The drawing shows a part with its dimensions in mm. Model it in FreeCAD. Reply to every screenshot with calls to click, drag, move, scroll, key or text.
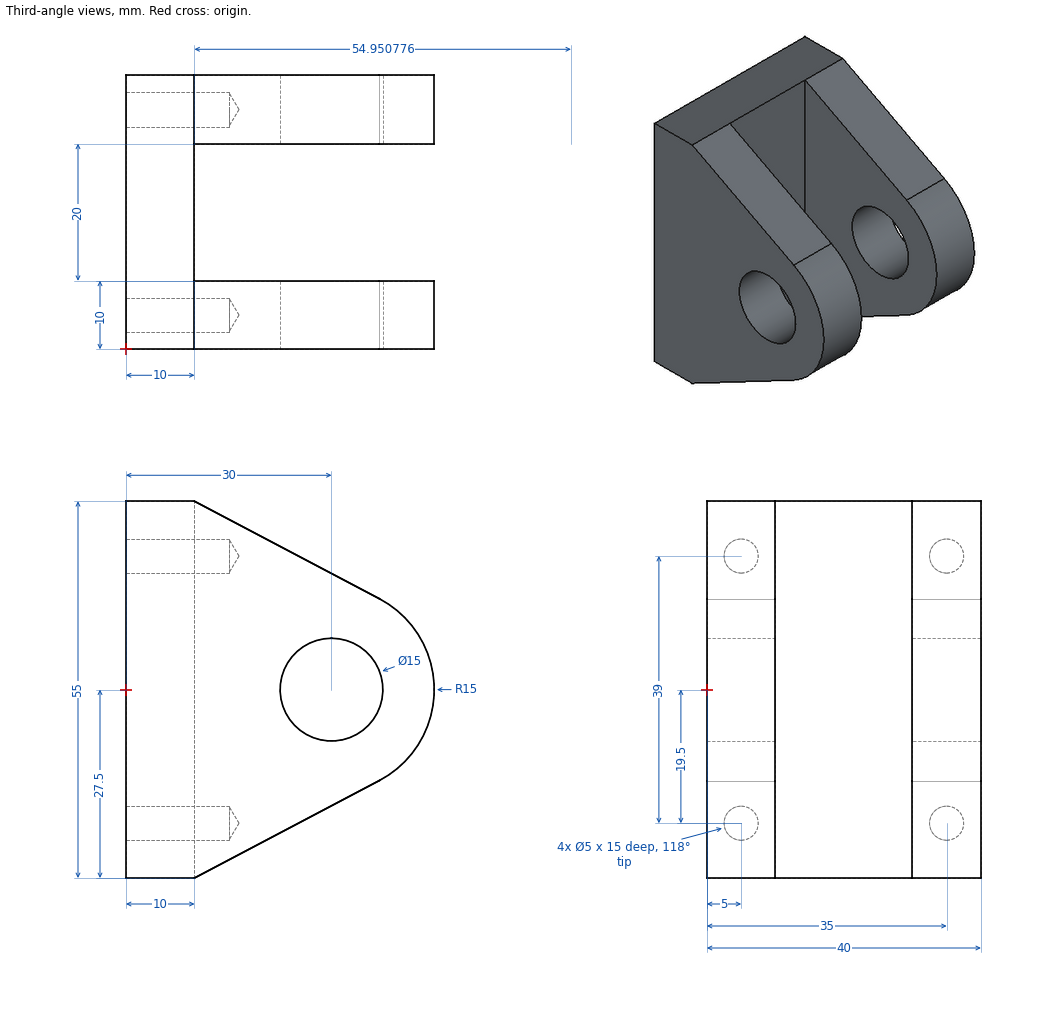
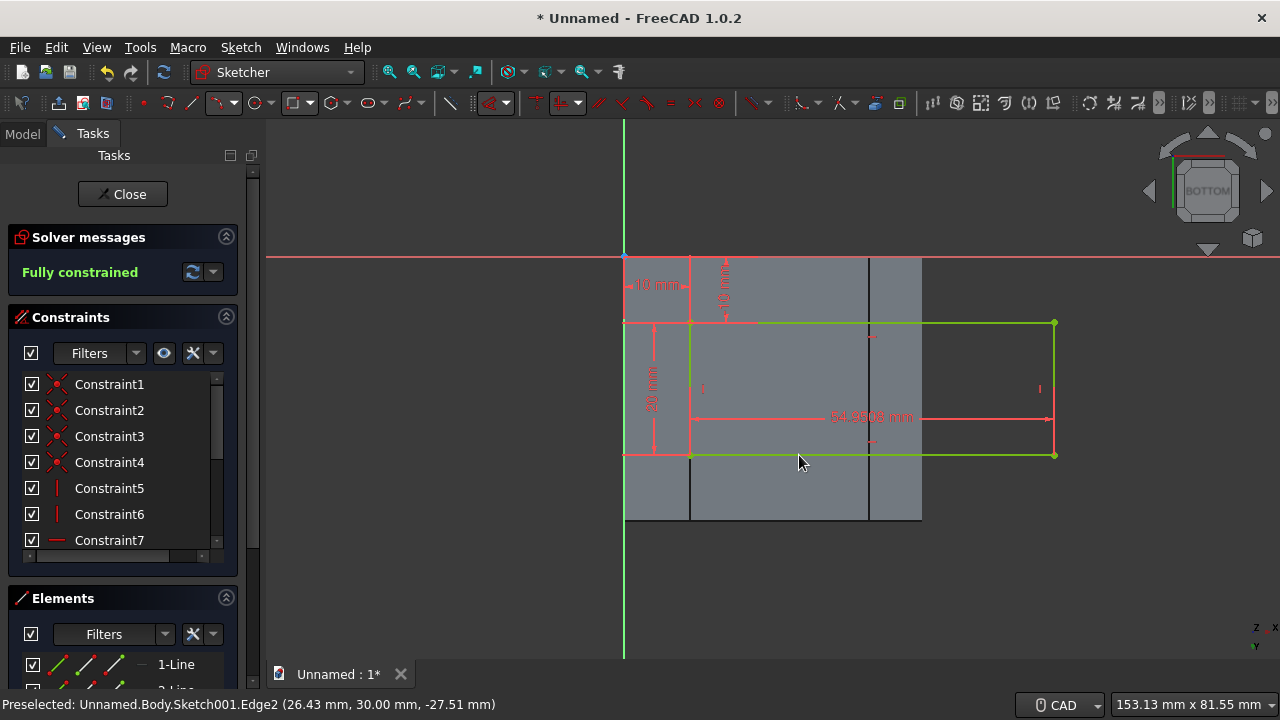
click(123, 194)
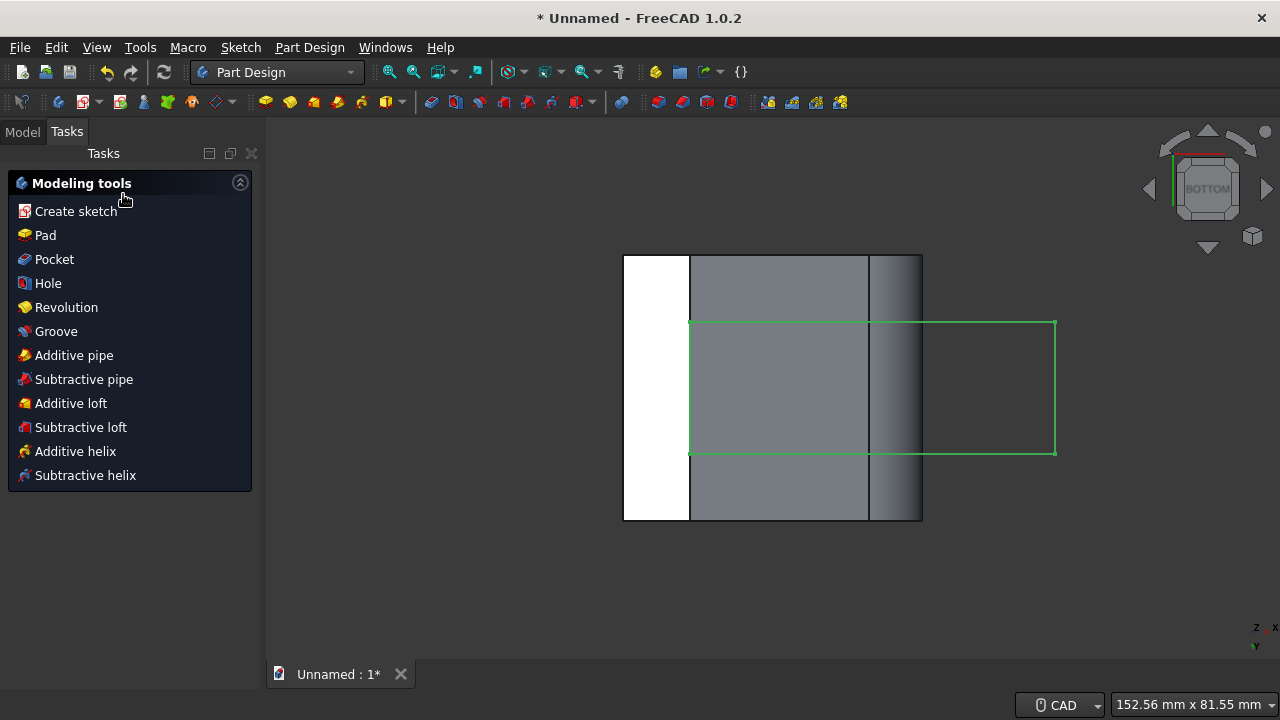
click(432, 102)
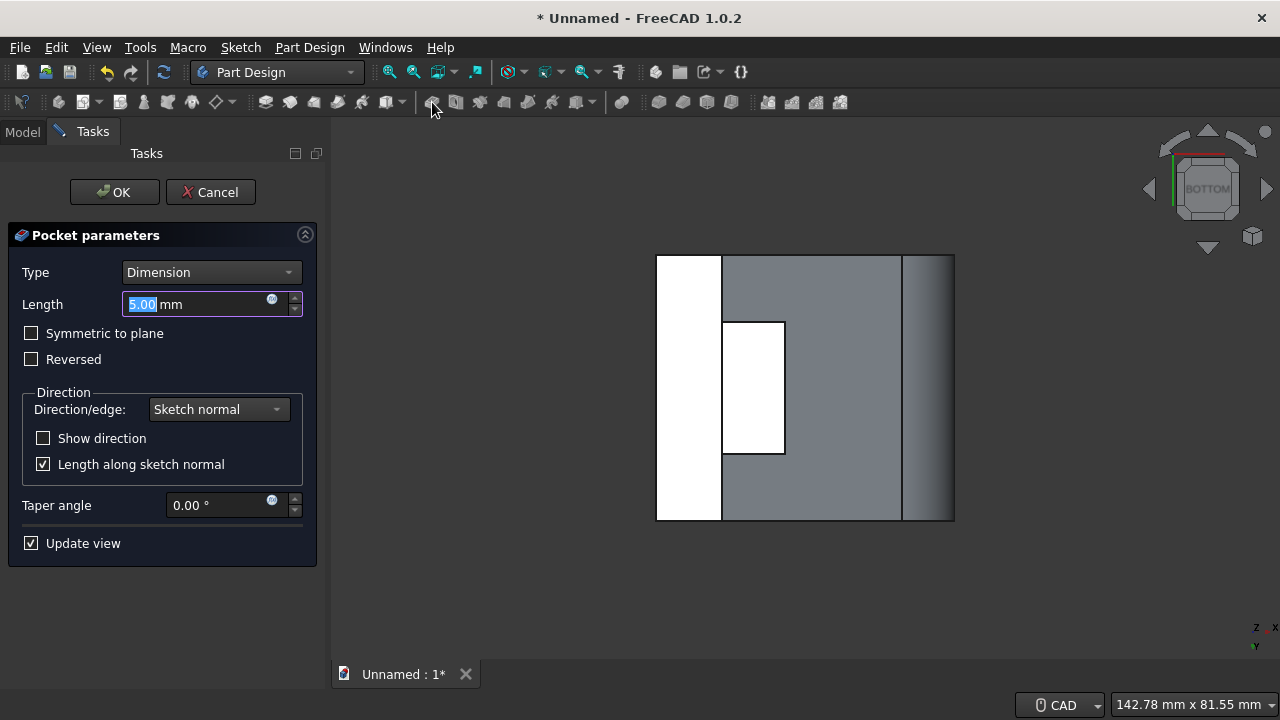
click(212, 272)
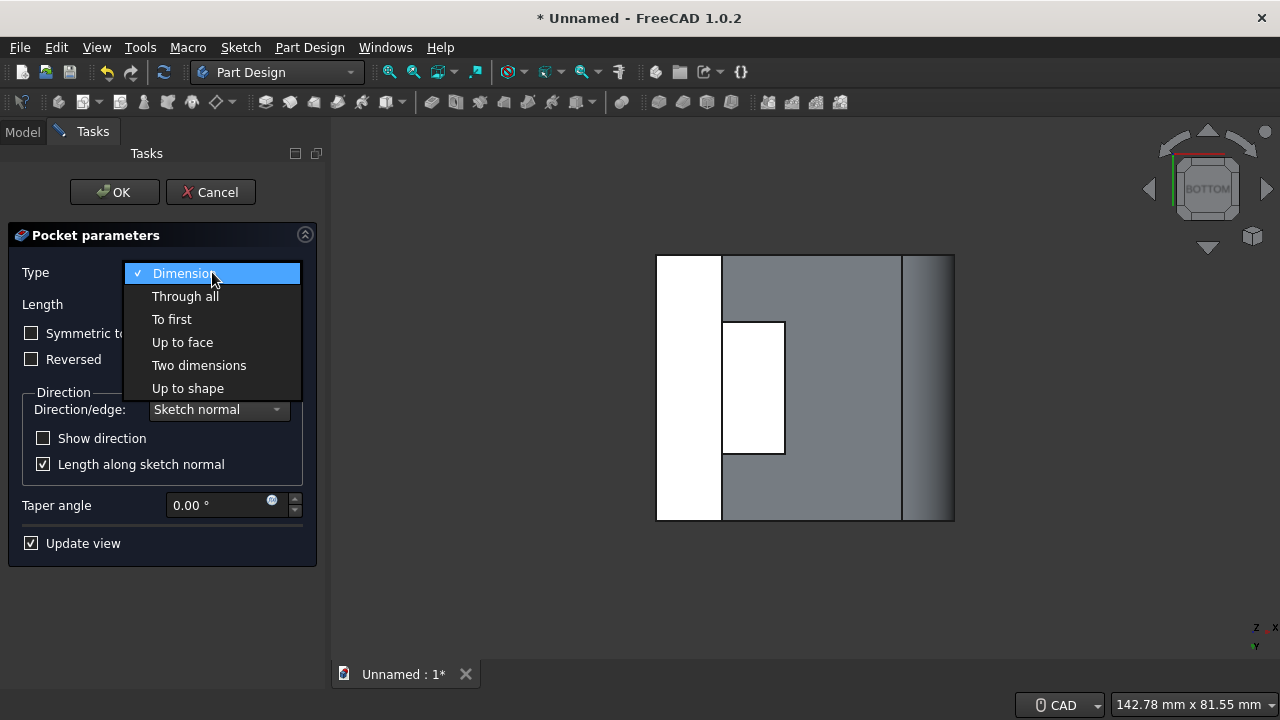
click(212, 296)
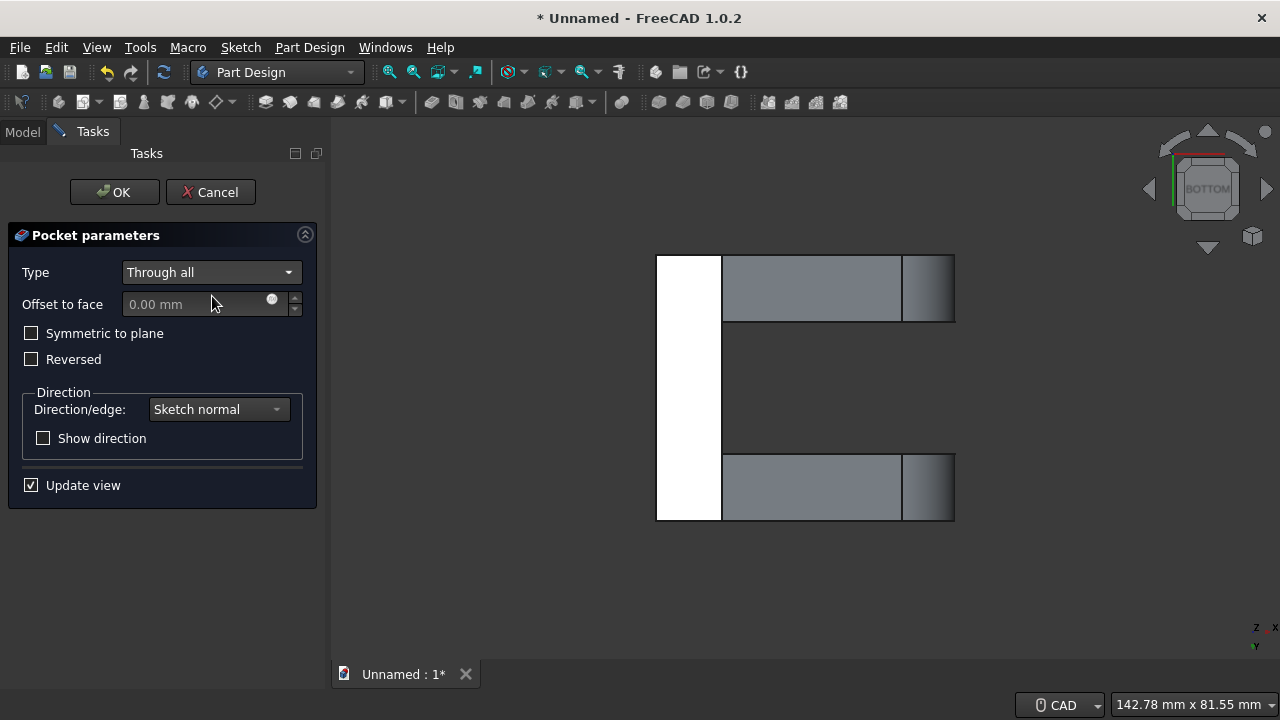
click(115, 192)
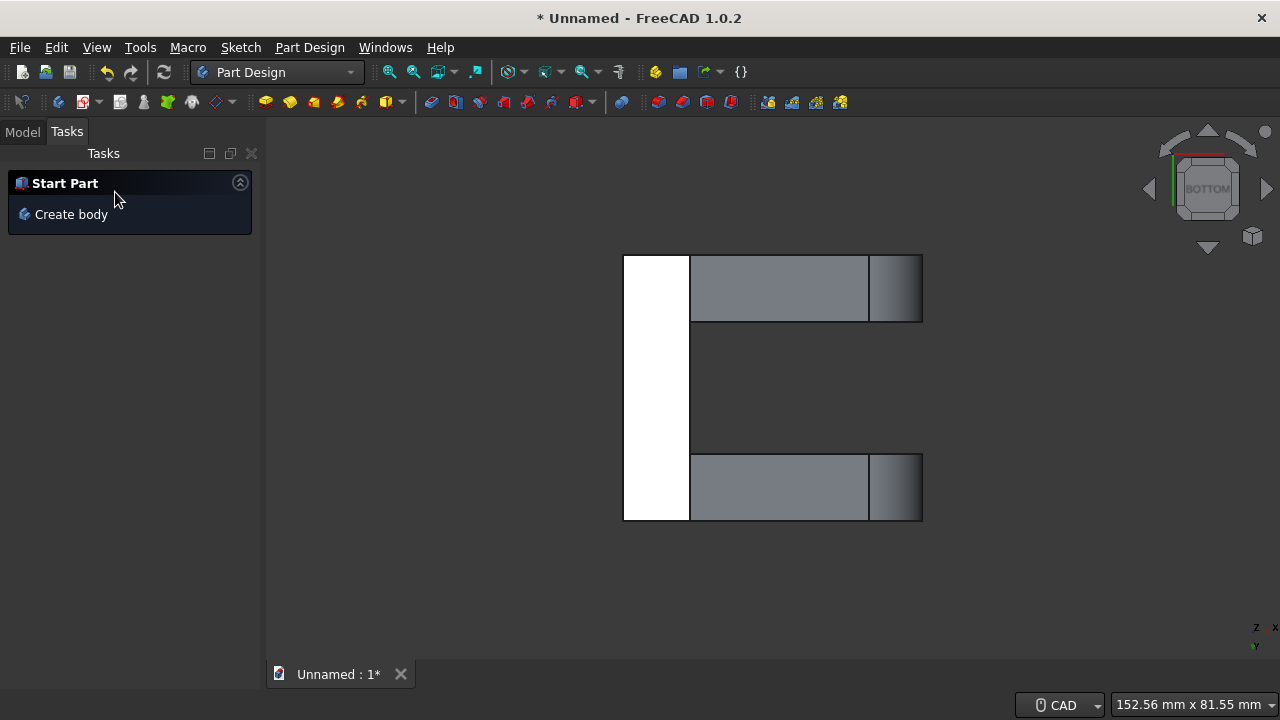
click(84, 102)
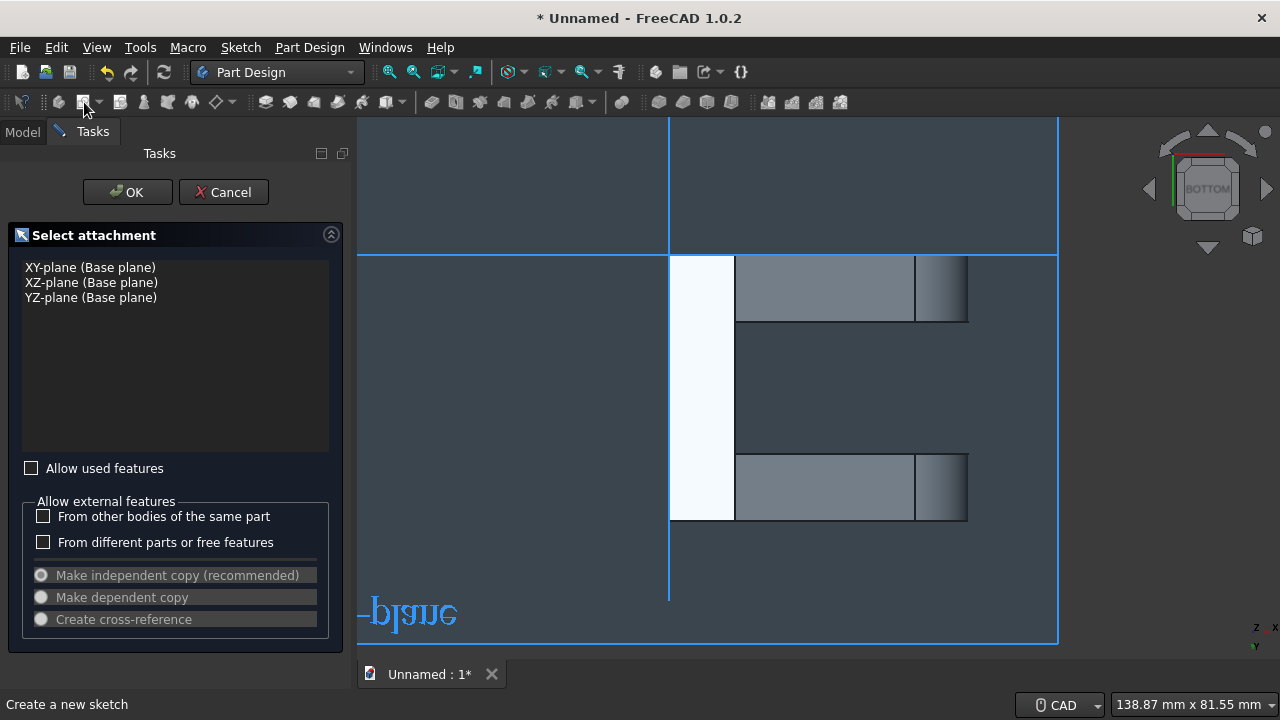
click(82, 298)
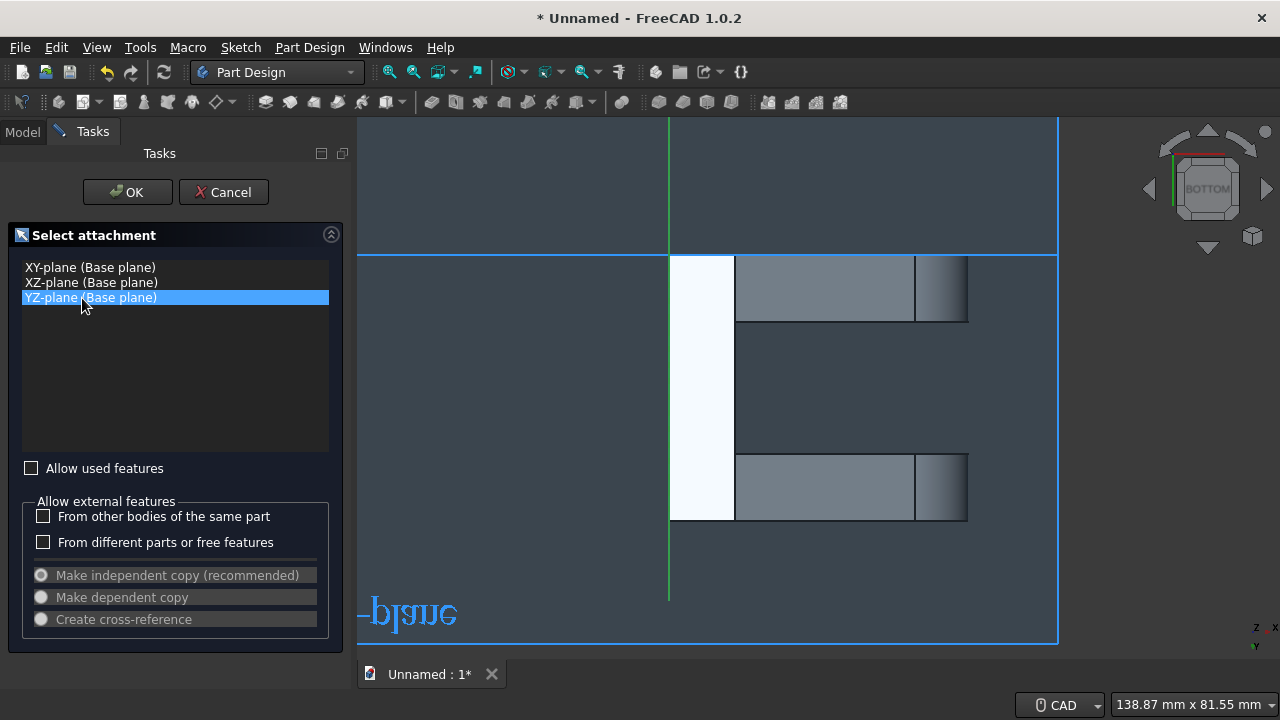
click(128, 192)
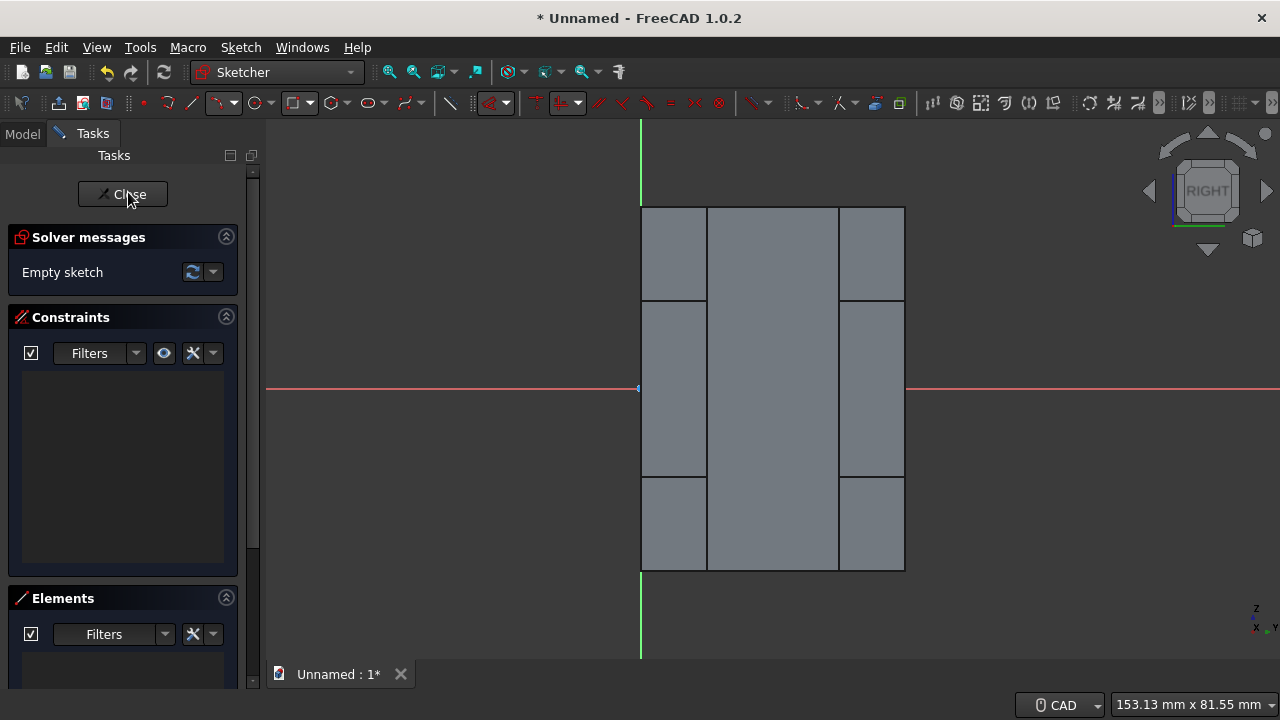
key(q)
key(s)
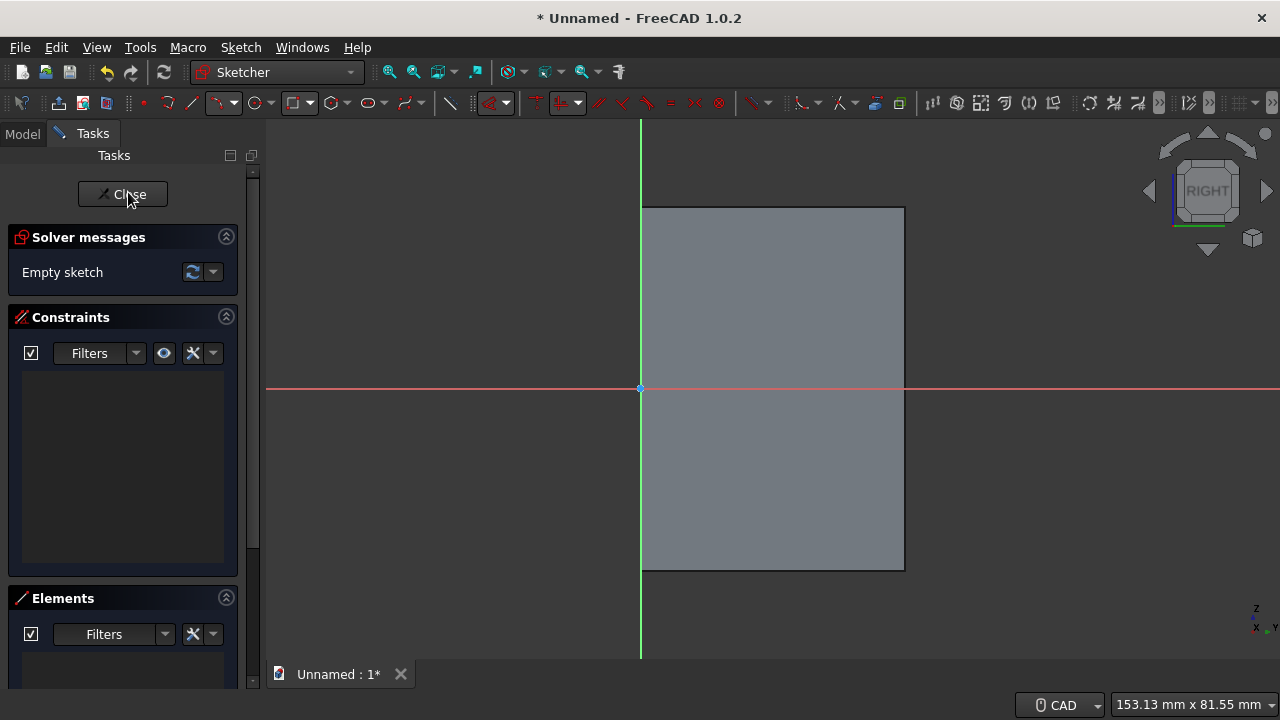
key(g)
key(c)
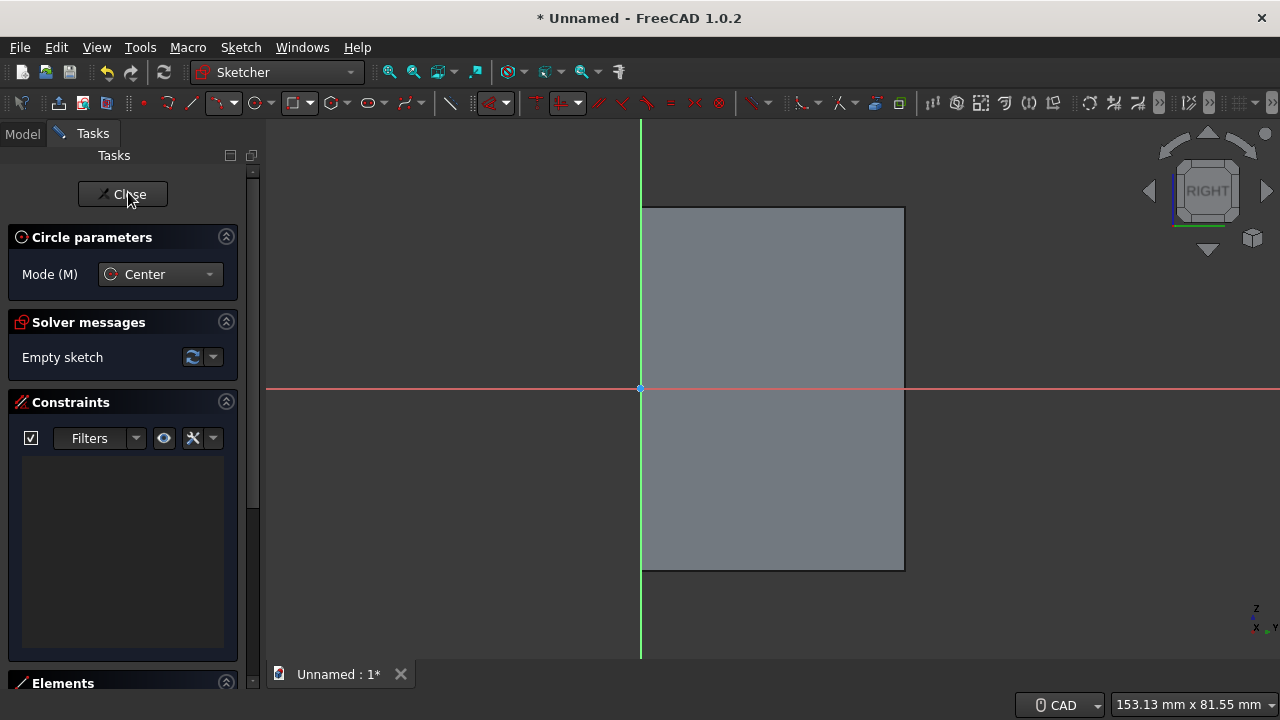
scroll(674, 518, up, 2)